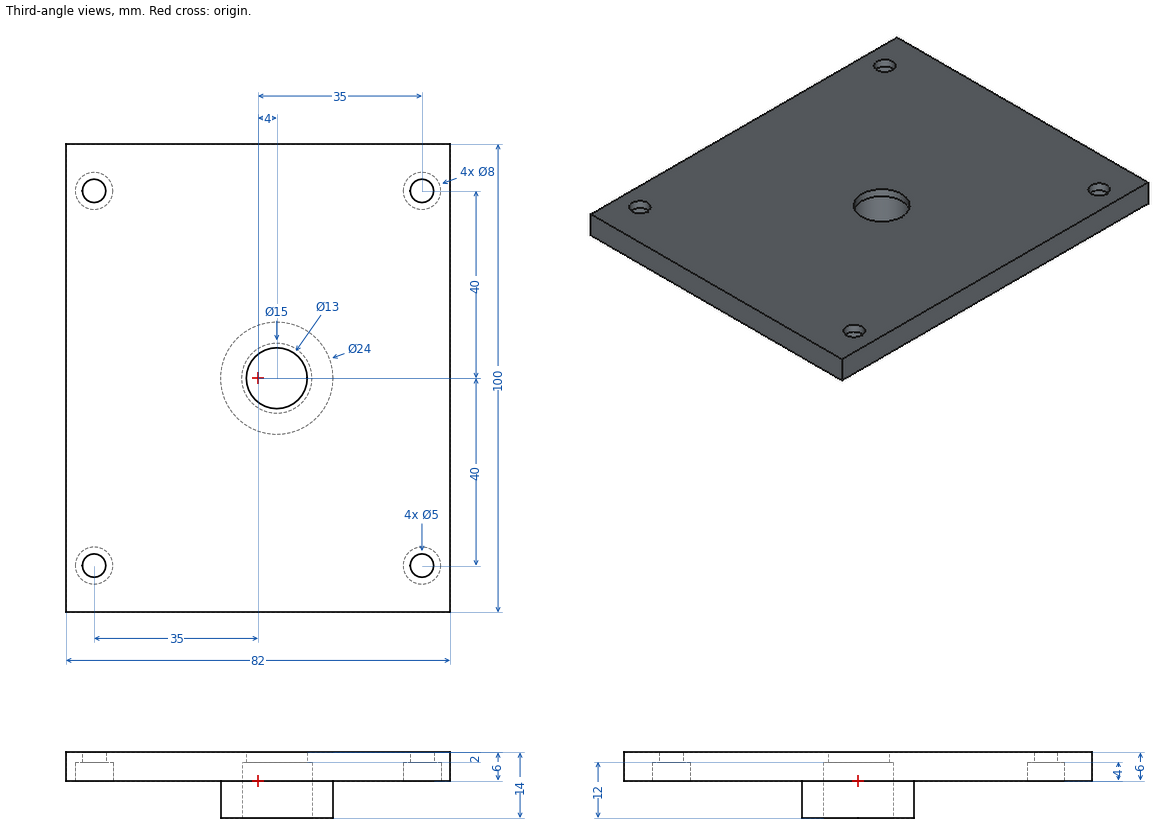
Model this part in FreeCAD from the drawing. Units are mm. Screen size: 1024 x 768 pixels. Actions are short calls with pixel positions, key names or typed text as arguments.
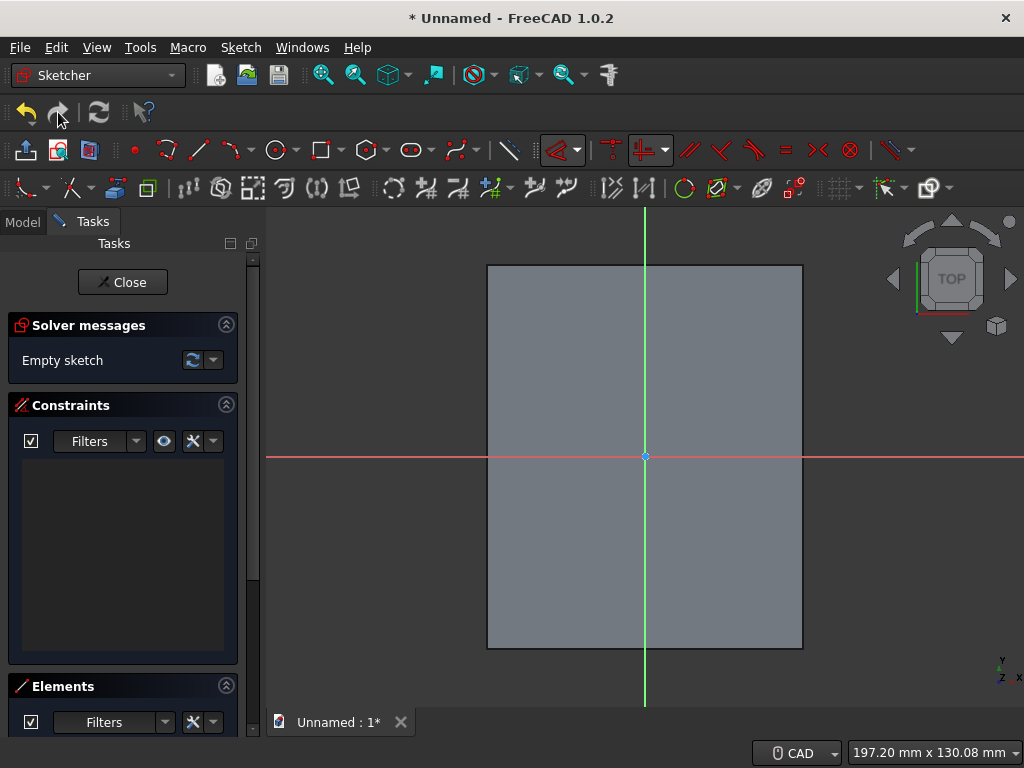
scroll(677, 457, up, 9)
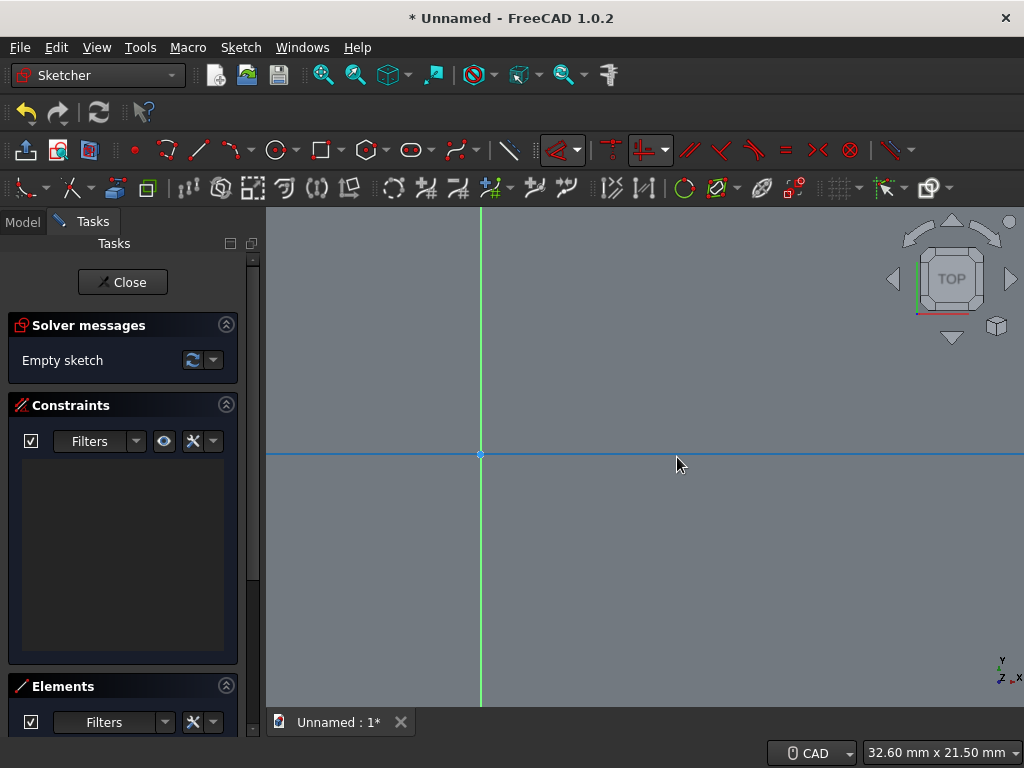
click(276, 150)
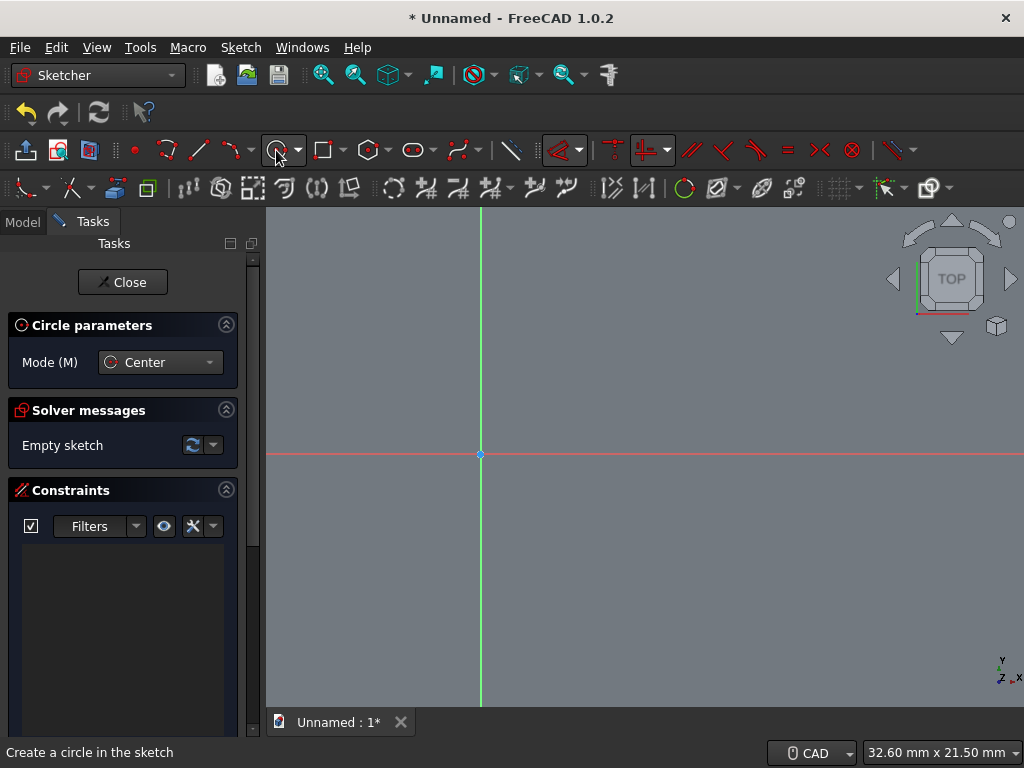
click(574, 454)
move(681, 348)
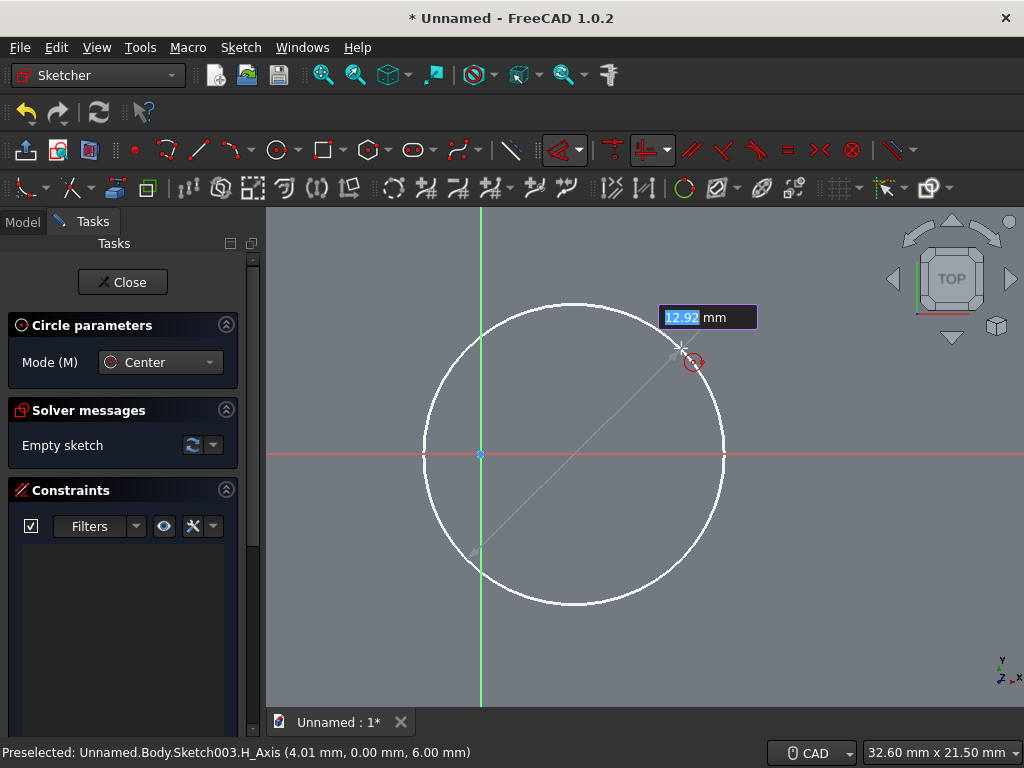
text(13)
key(Return)
key(Escape)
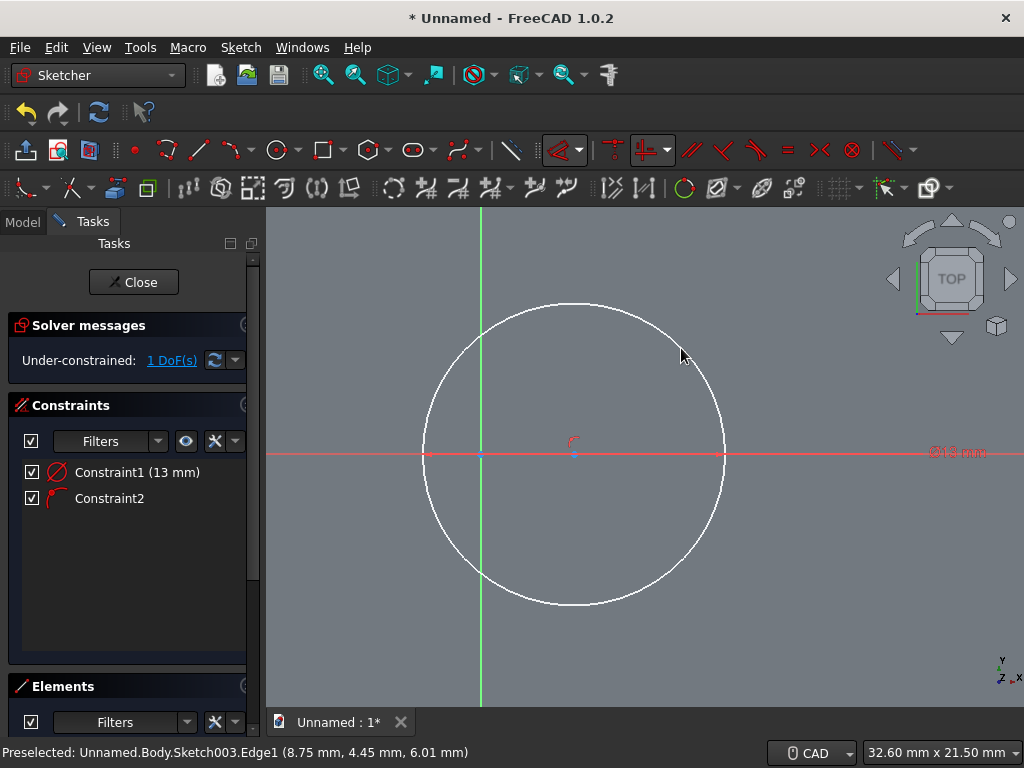
click(574, 454)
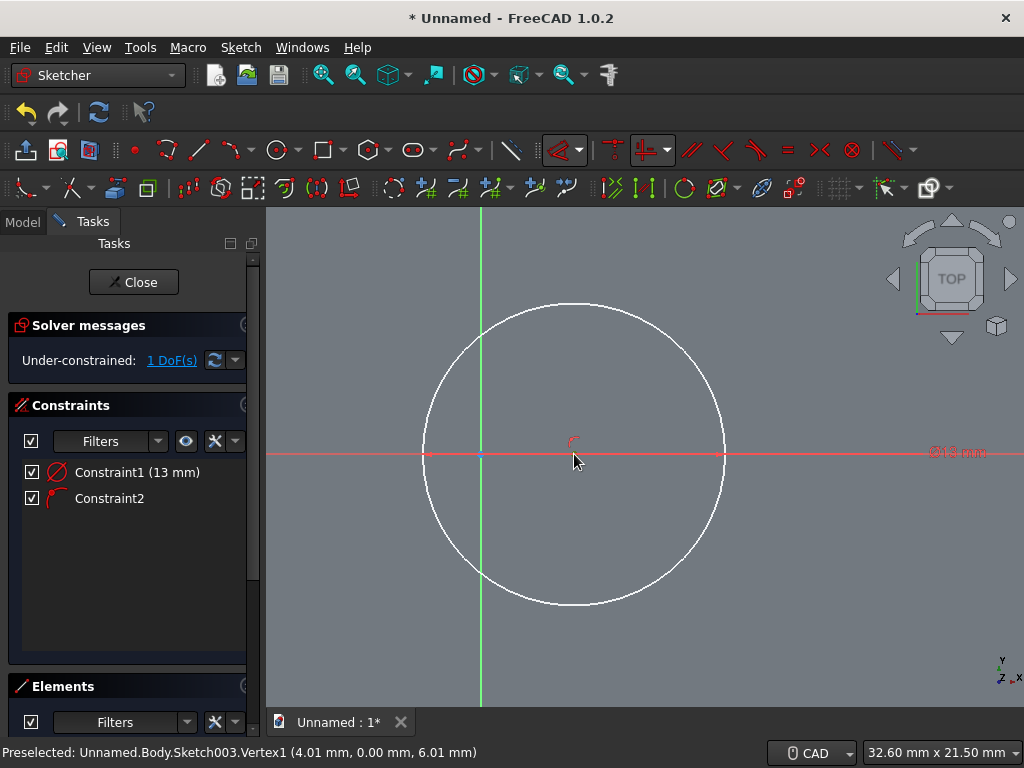
key(l)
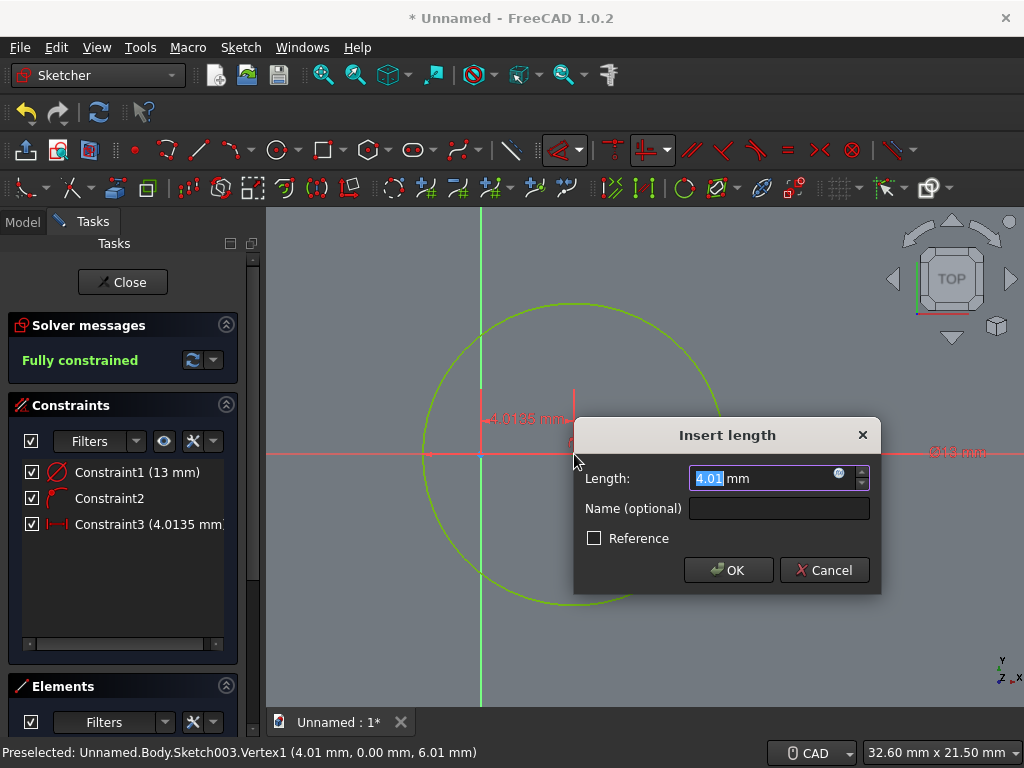
text(4)
key(Return)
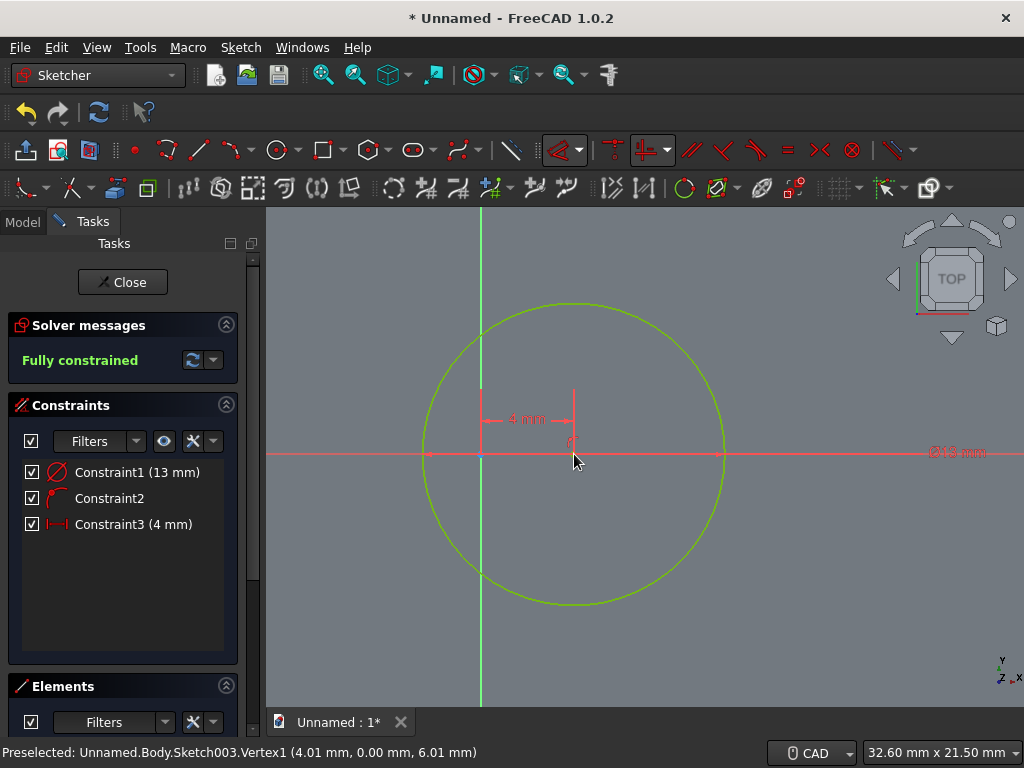
click(123, 282)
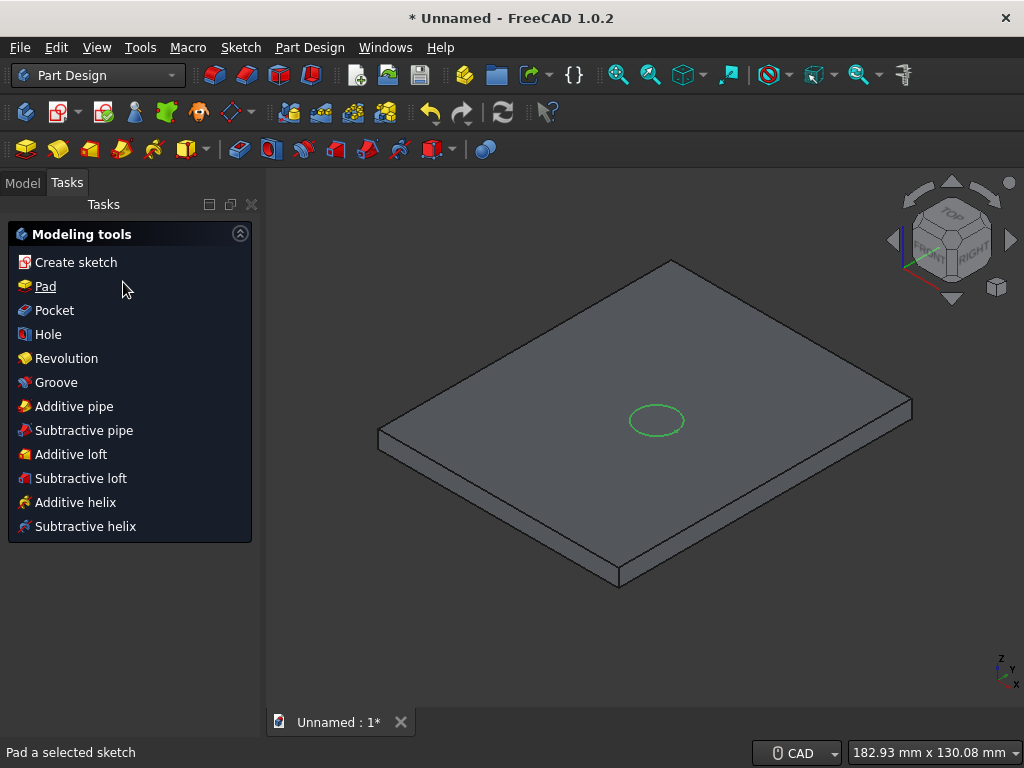
click(240, 150)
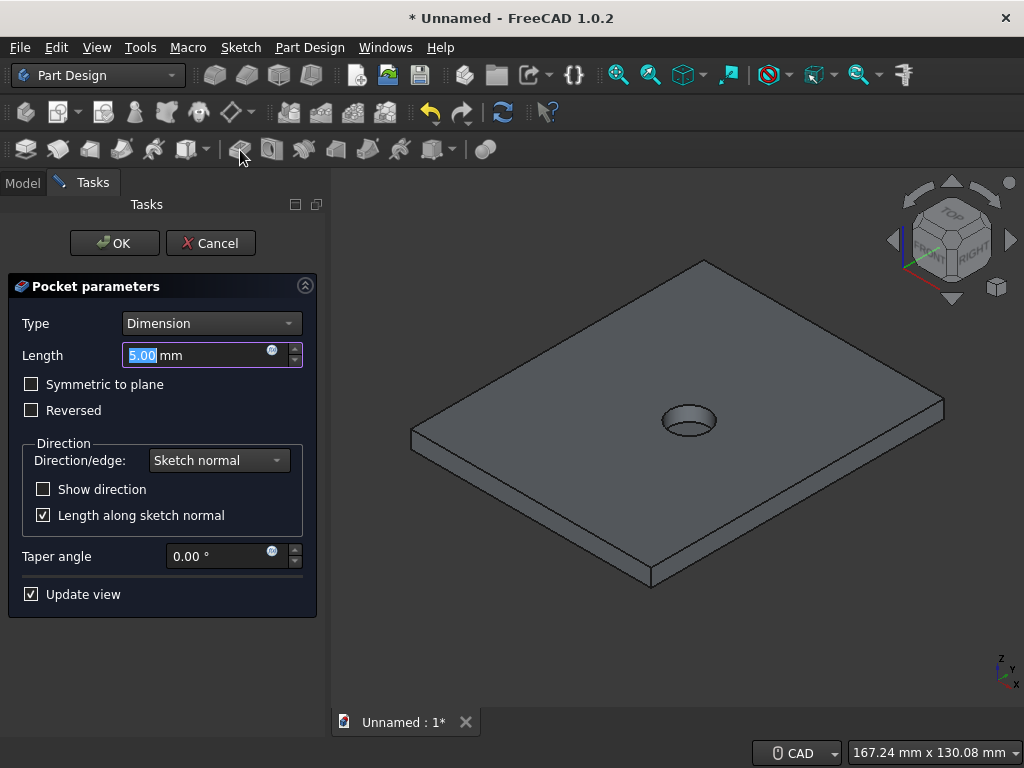
text(2)
key(Tab)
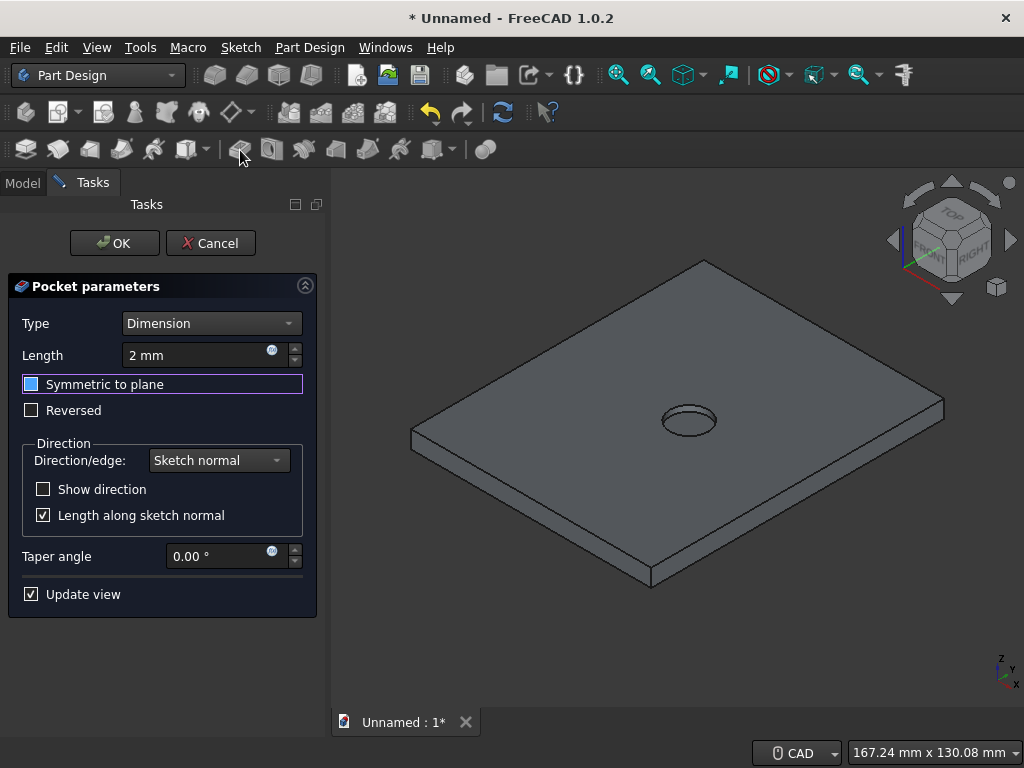
click(115, 243)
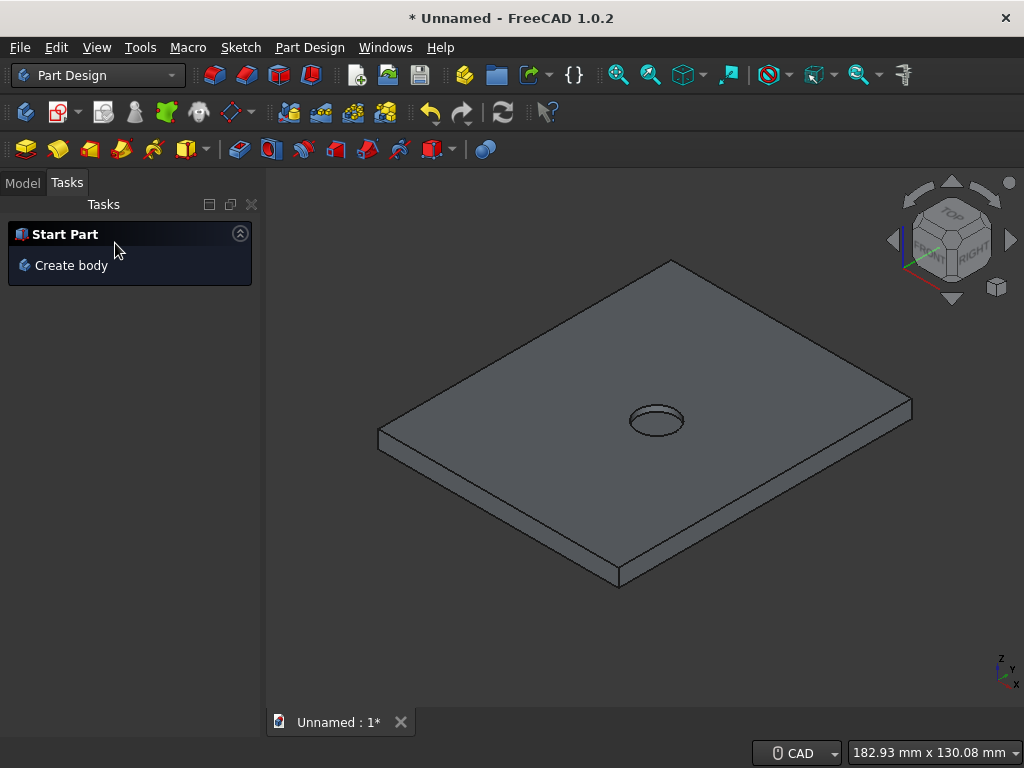
key(5)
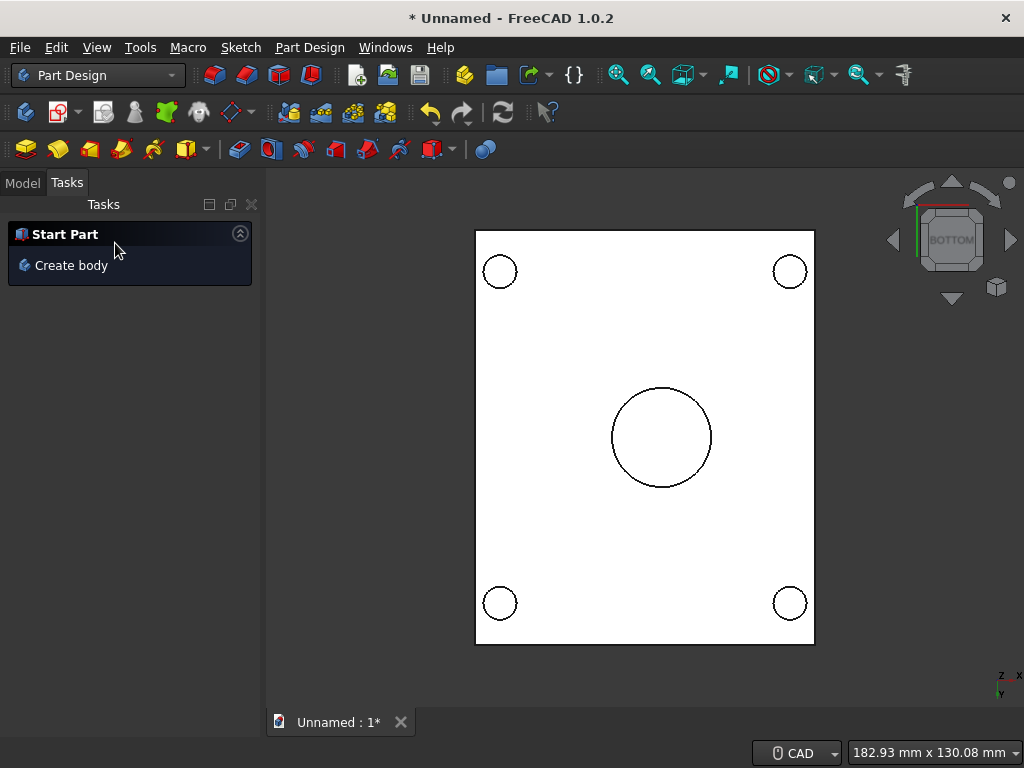
click(662, 437)